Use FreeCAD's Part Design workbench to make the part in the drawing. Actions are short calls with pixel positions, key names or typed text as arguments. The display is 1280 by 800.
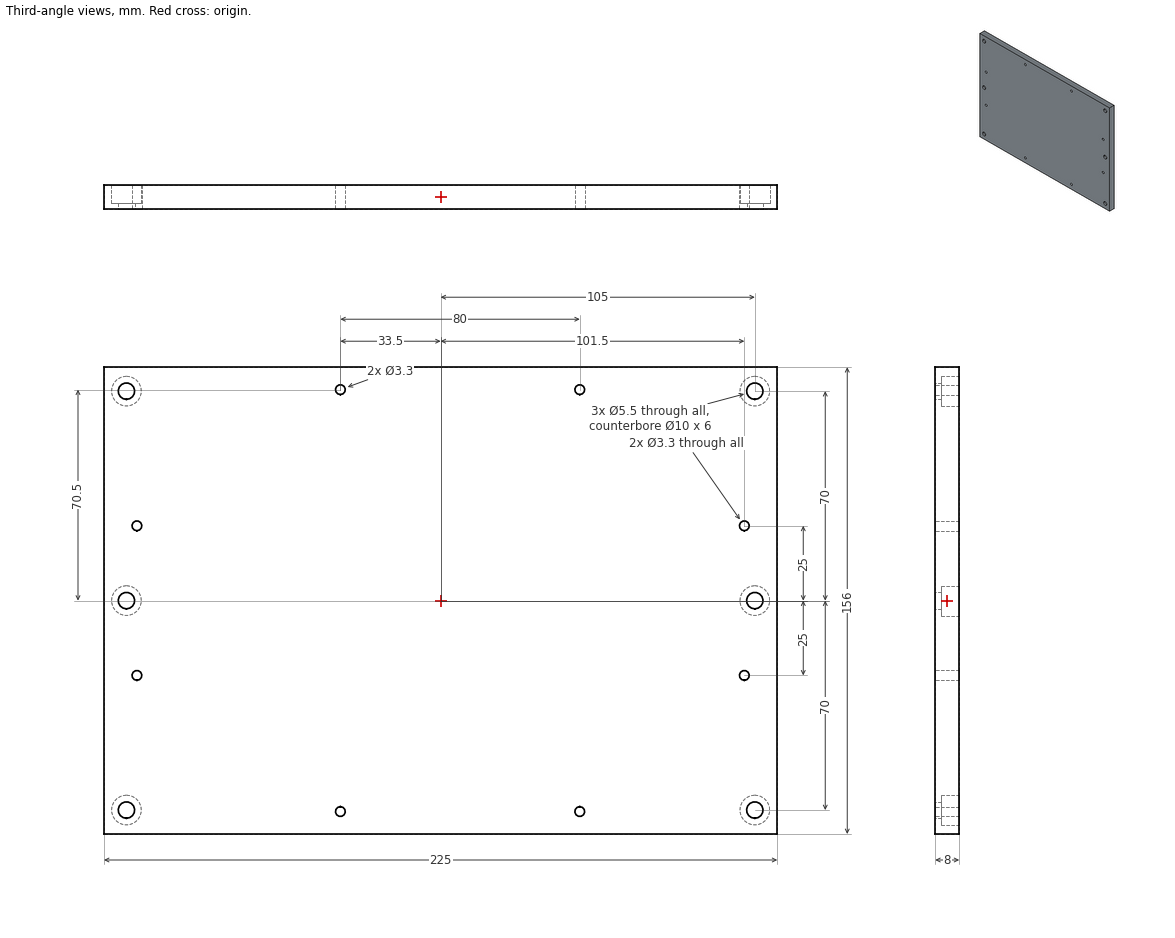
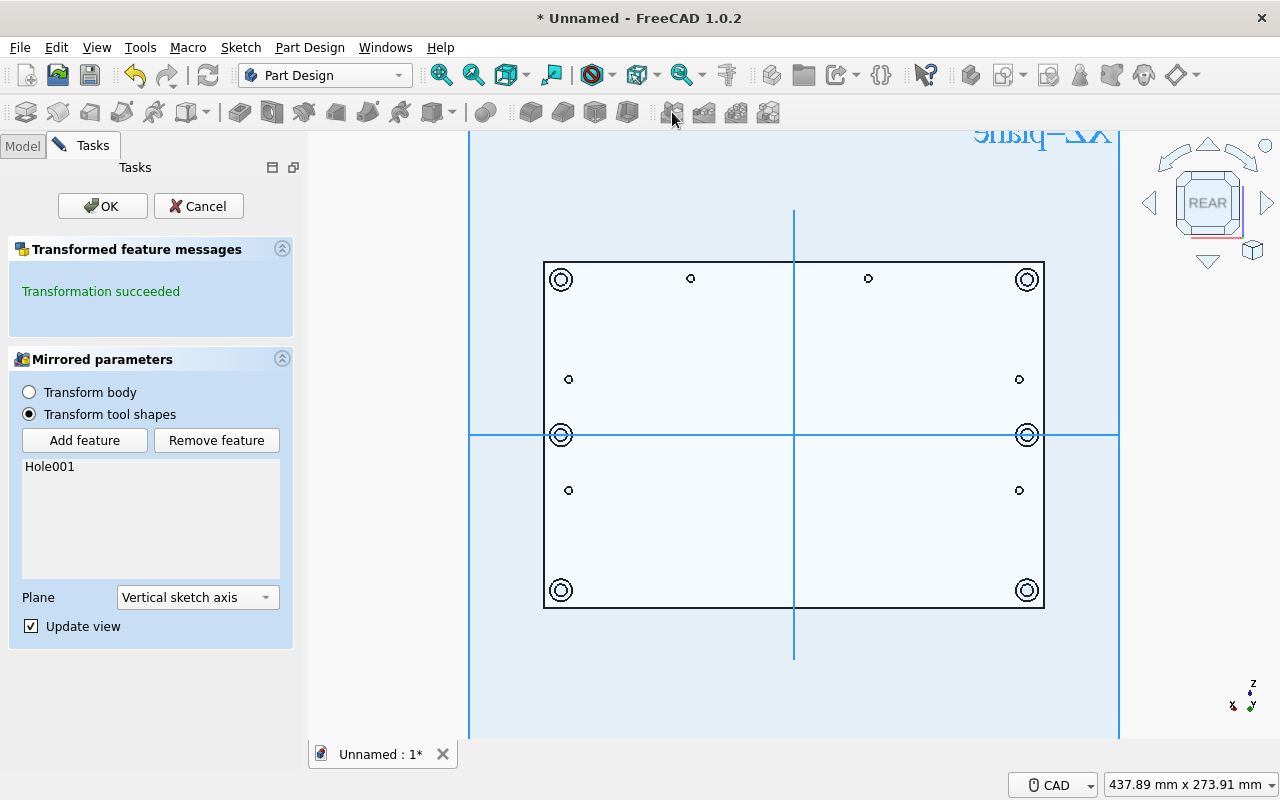
click(198, 598)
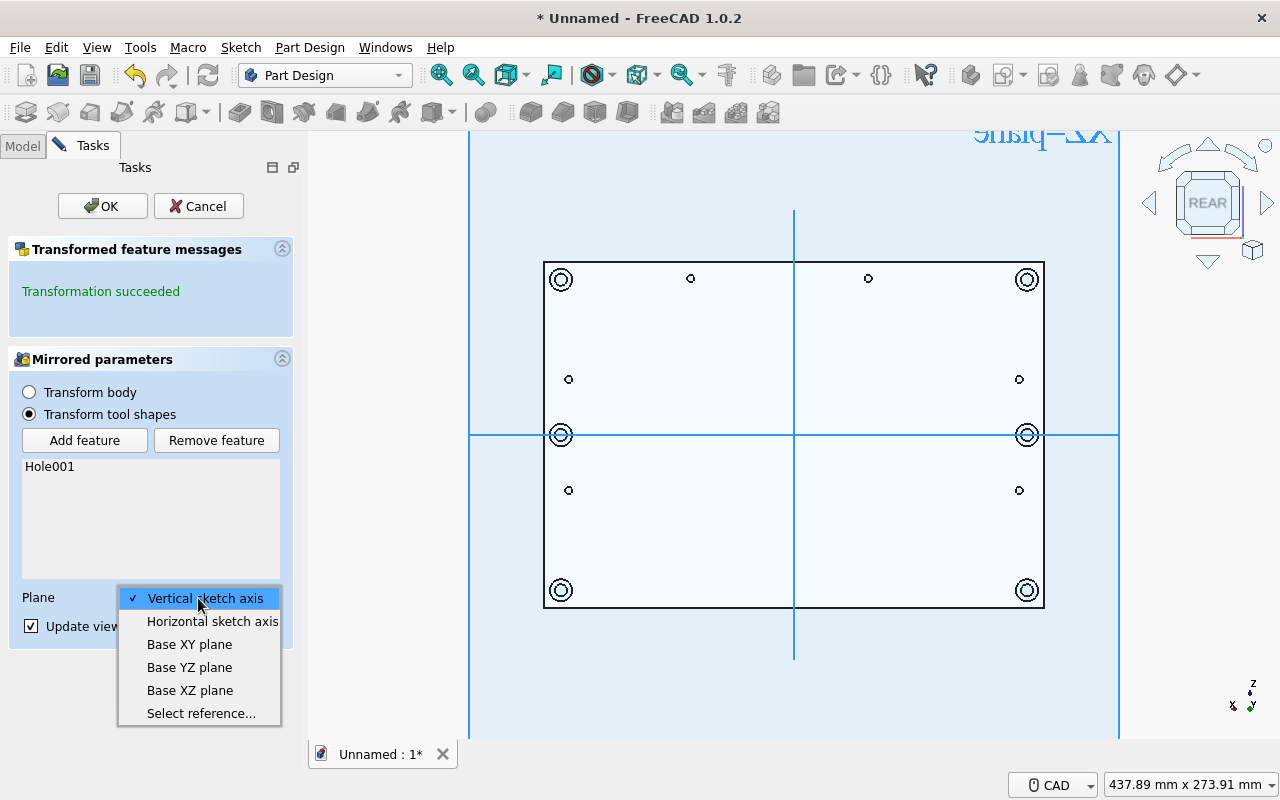
click(198, 668)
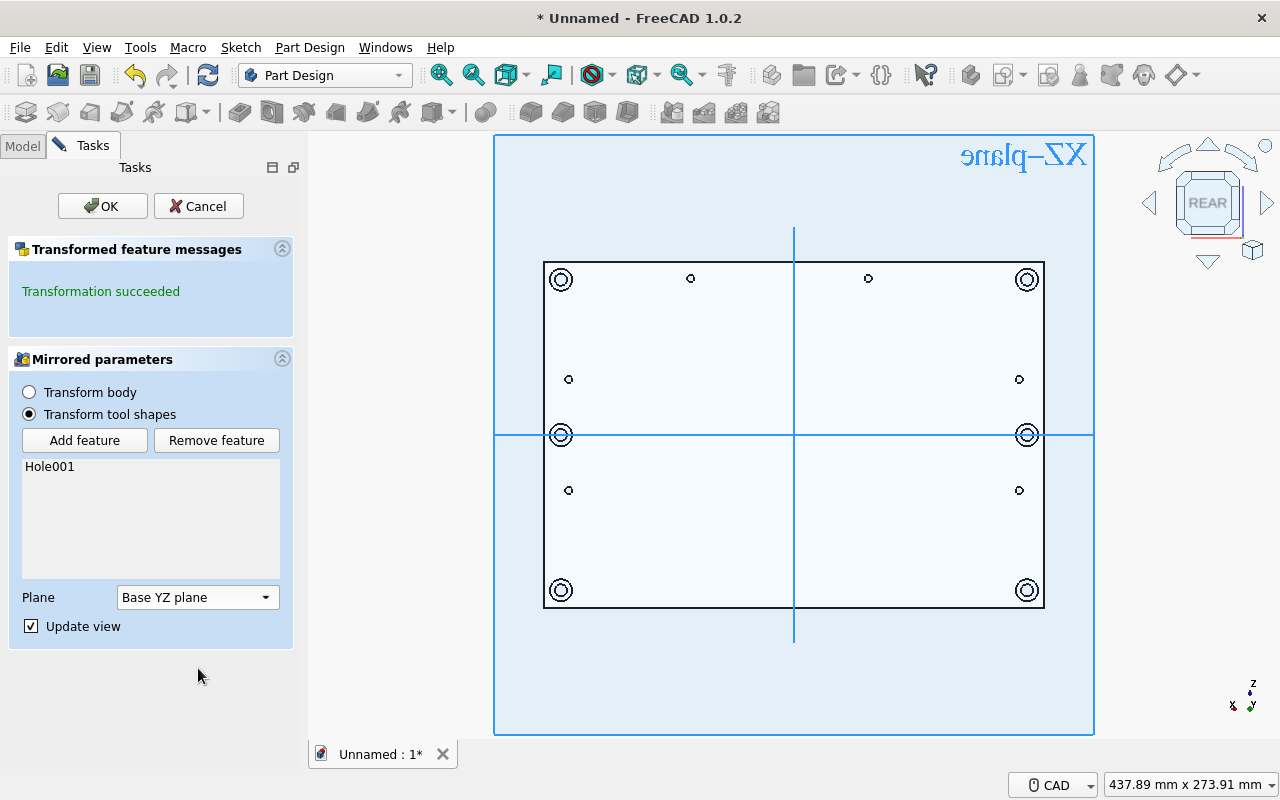
click(103, 206)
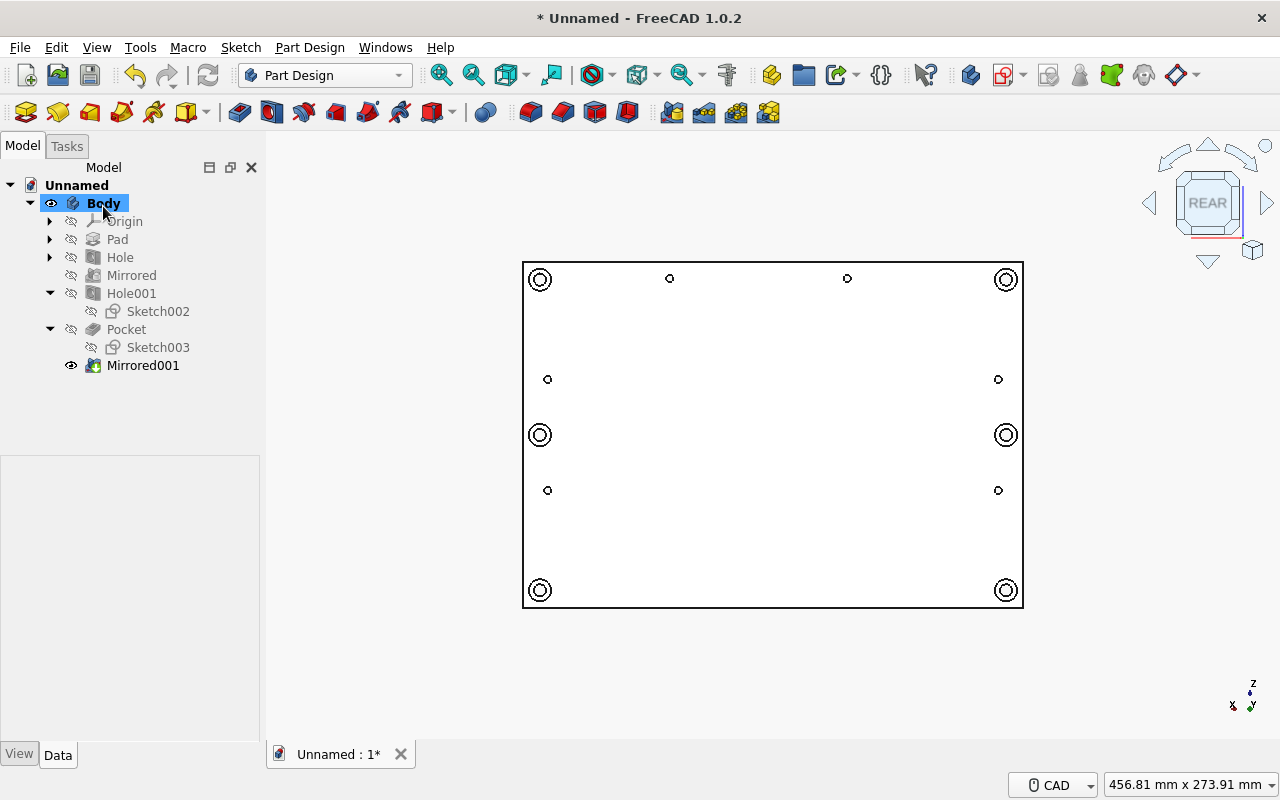
click(116, 329)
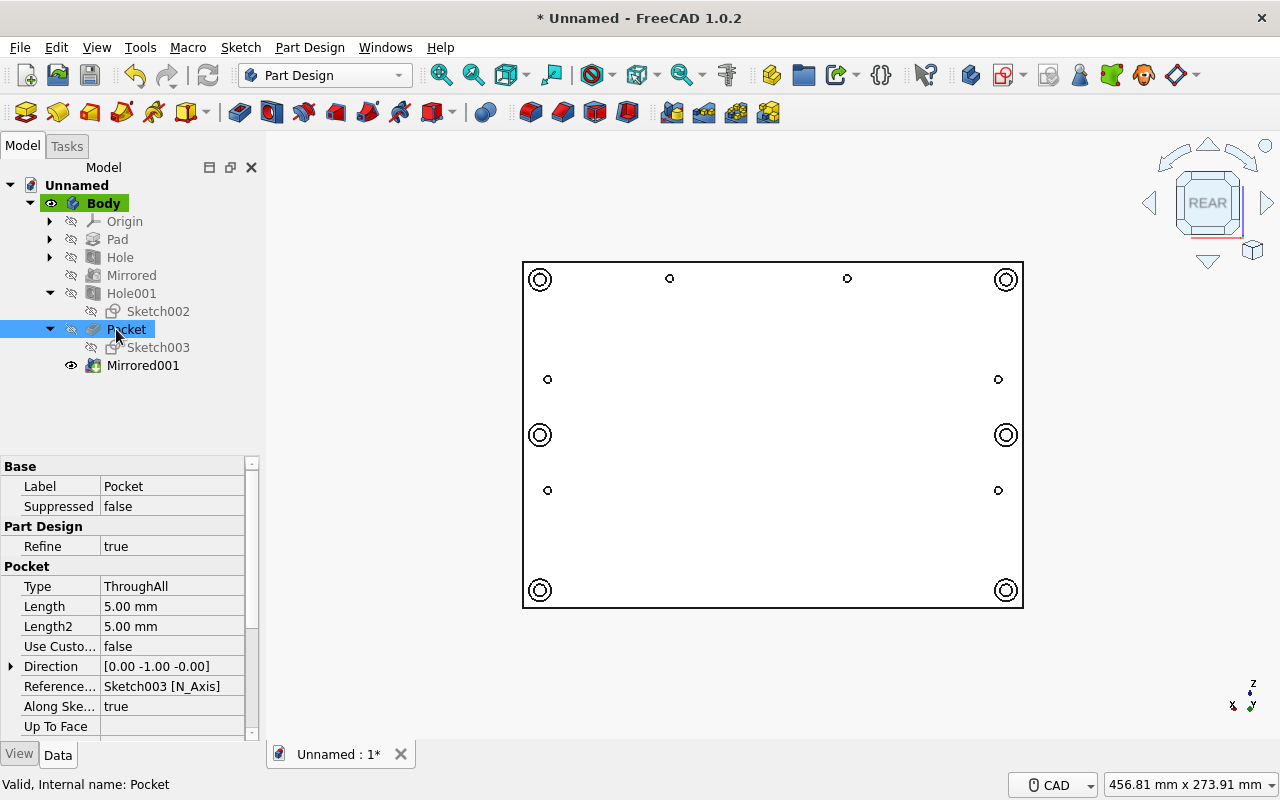
click(672, 112)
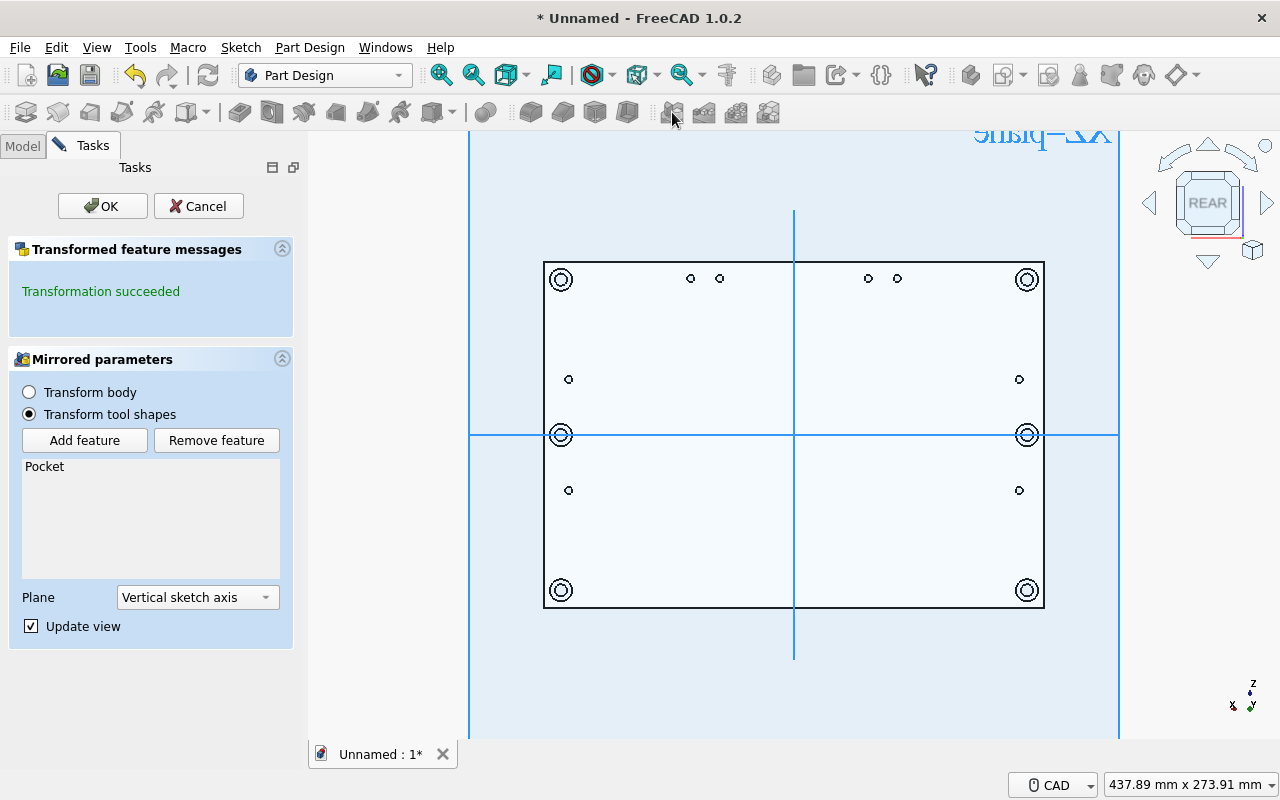
click(198, 598)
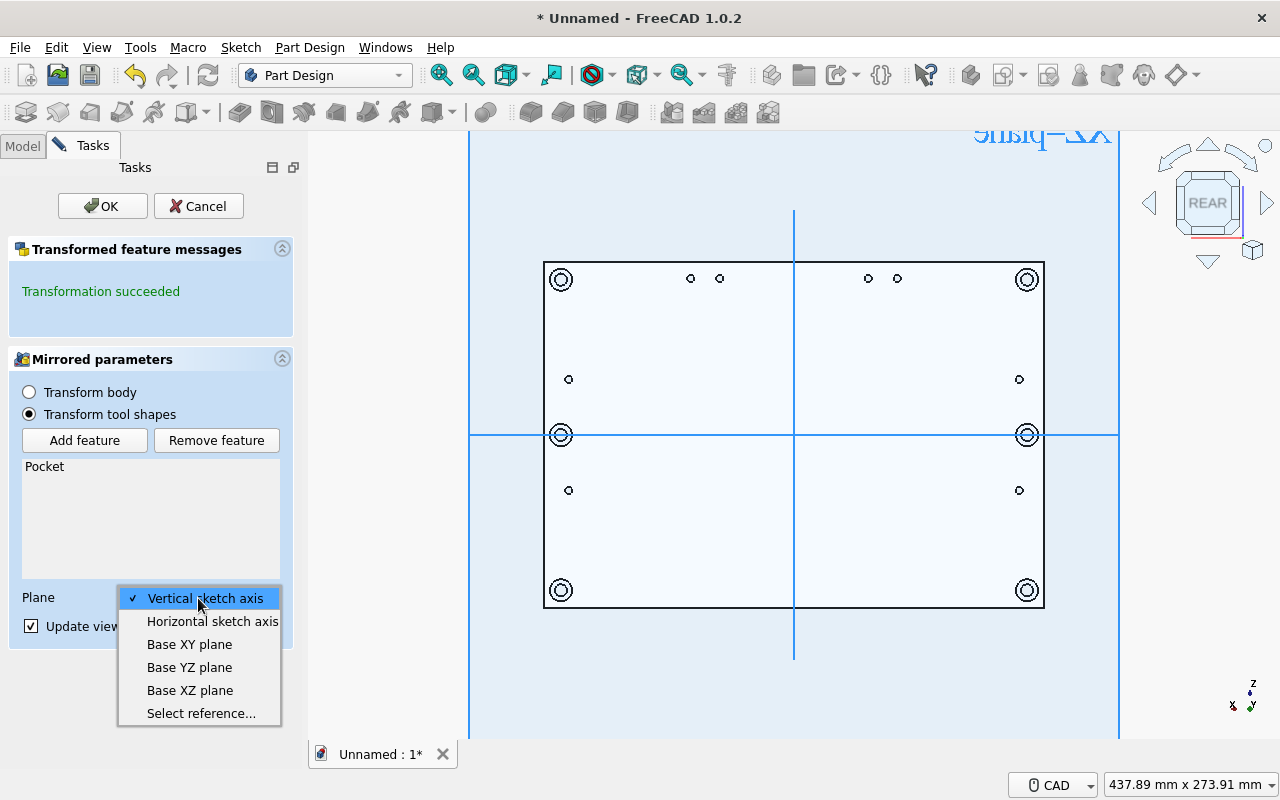
click(198, 644)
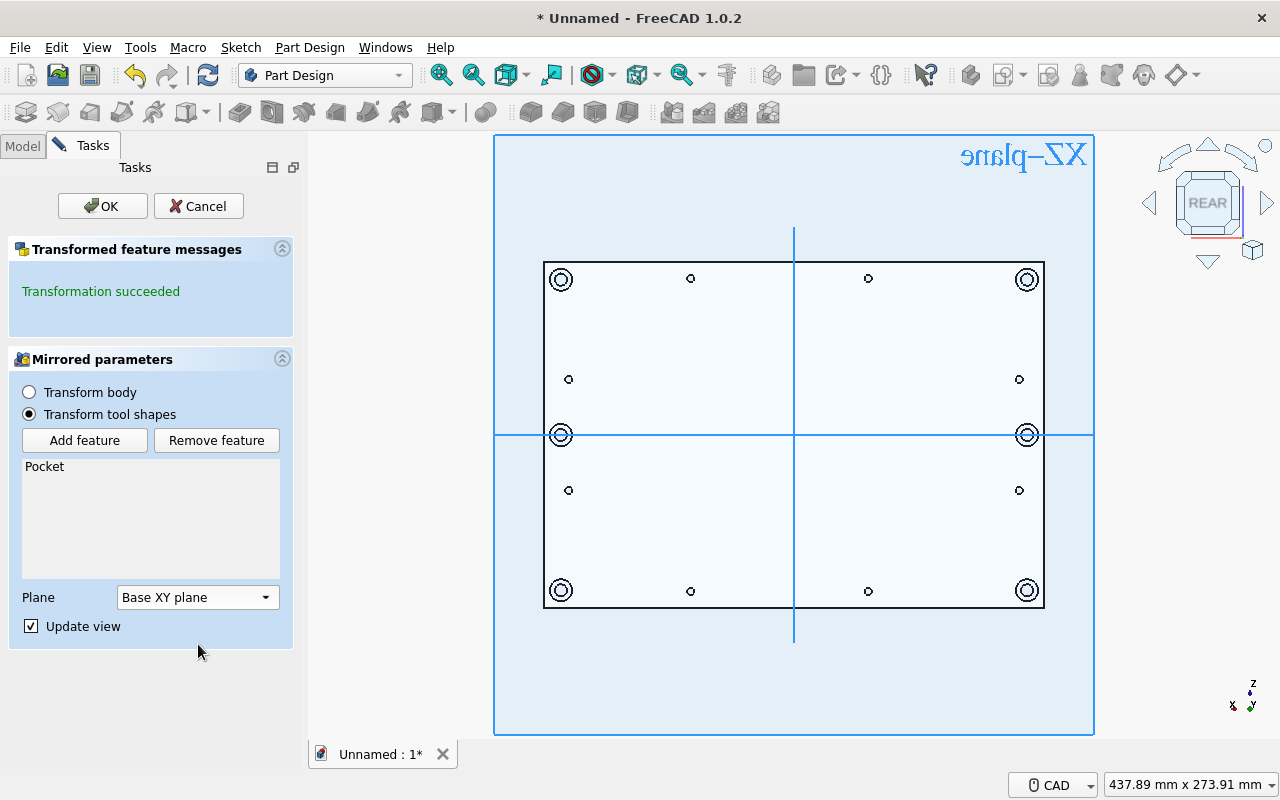
click(103, 206)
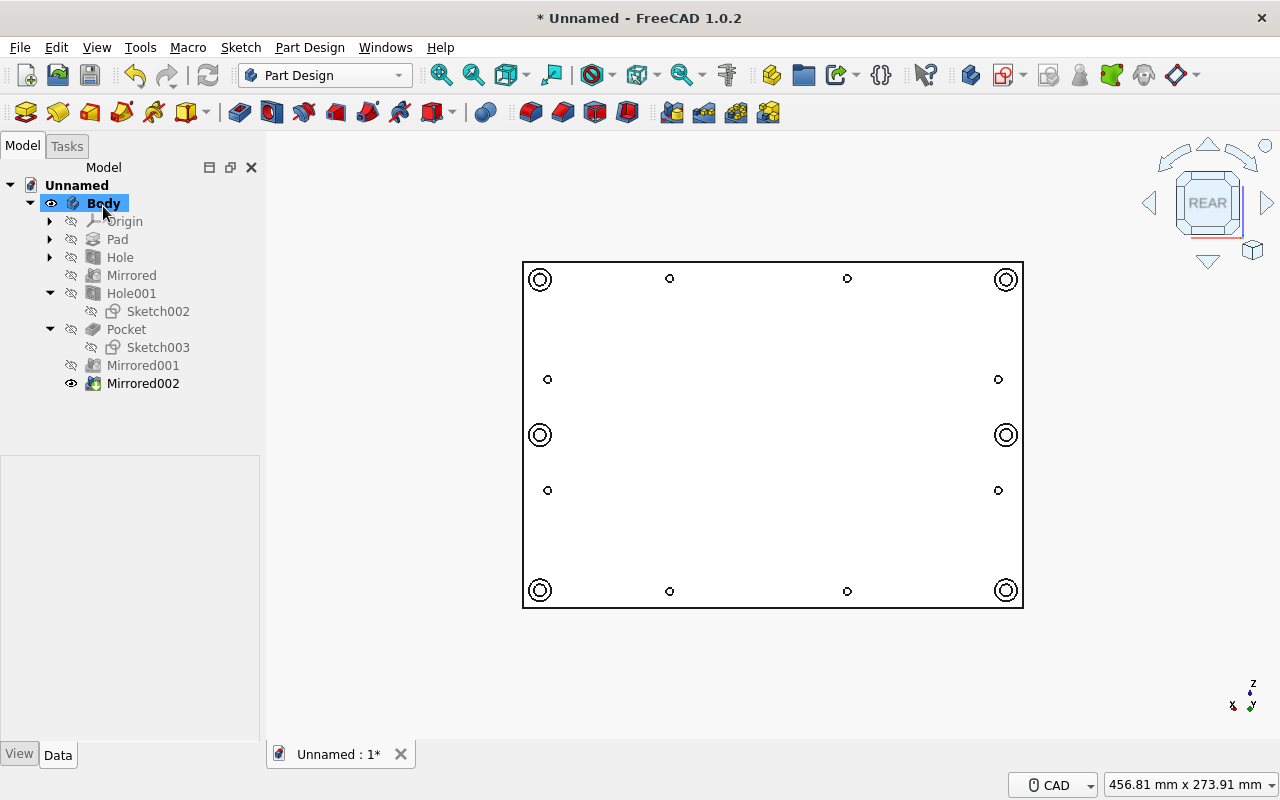
key(0)